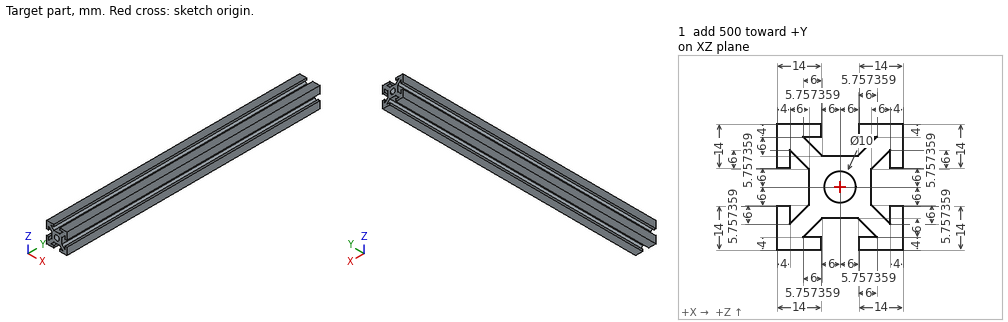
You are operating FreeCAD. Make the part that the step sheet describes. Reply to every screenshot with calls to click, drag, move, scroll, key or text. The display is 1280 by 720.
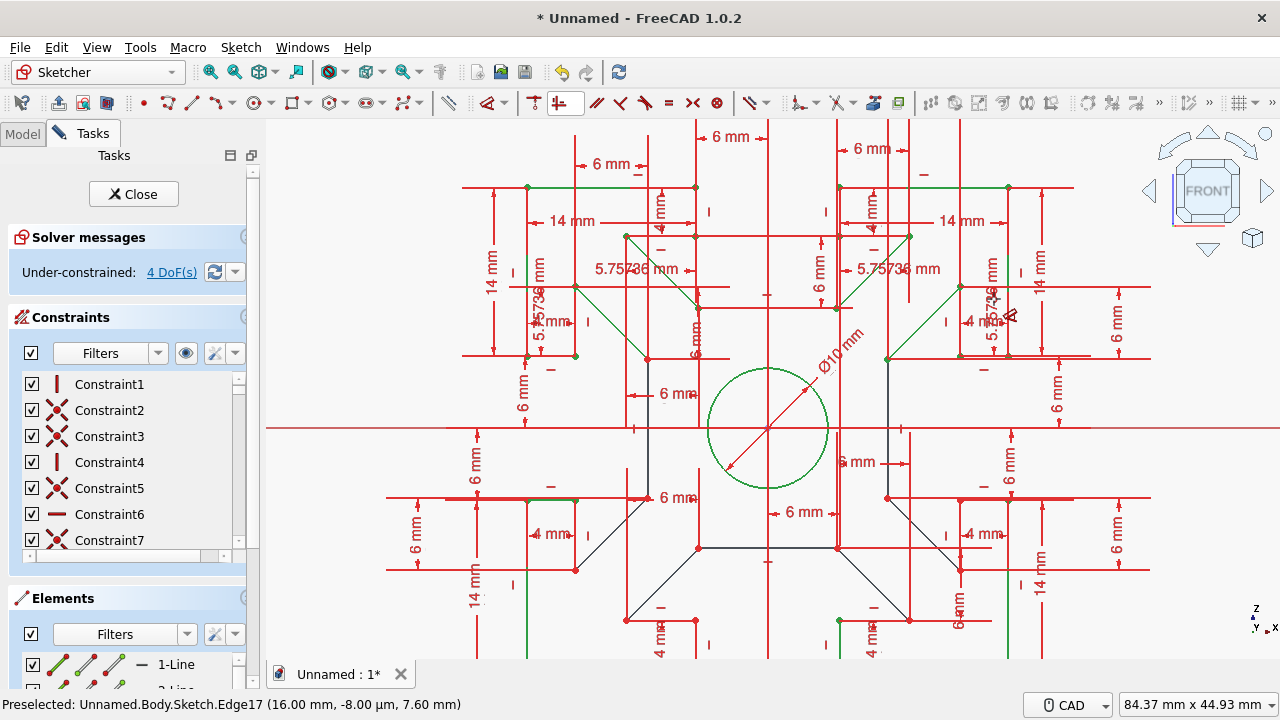
click(960, 549)
click(926, 511)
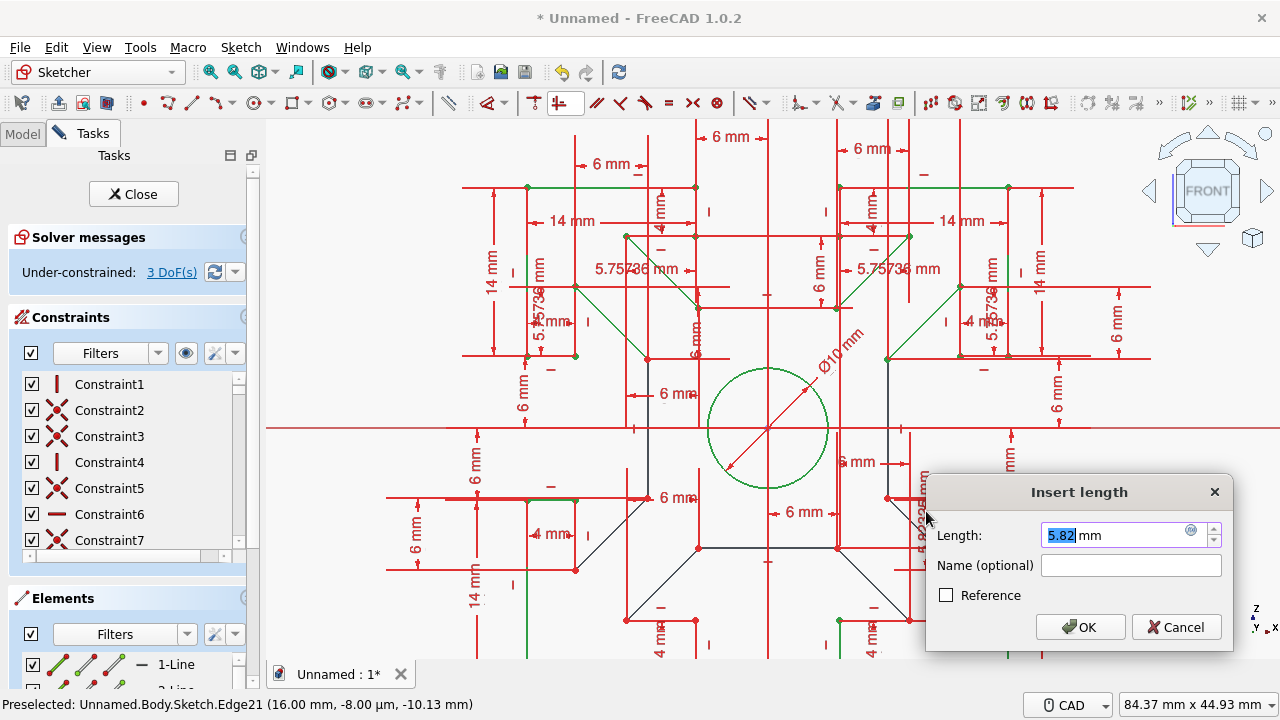
text(5.757359)
key(Return)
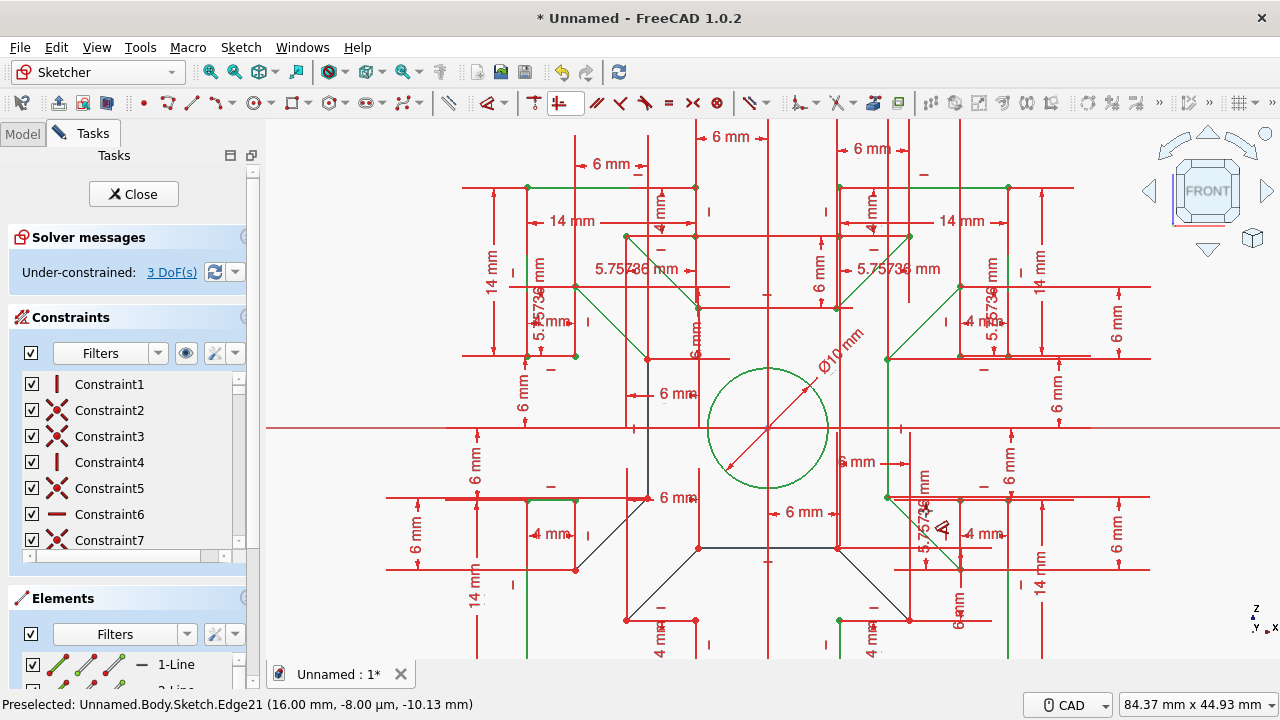
click(861, 621)
click(850, 587)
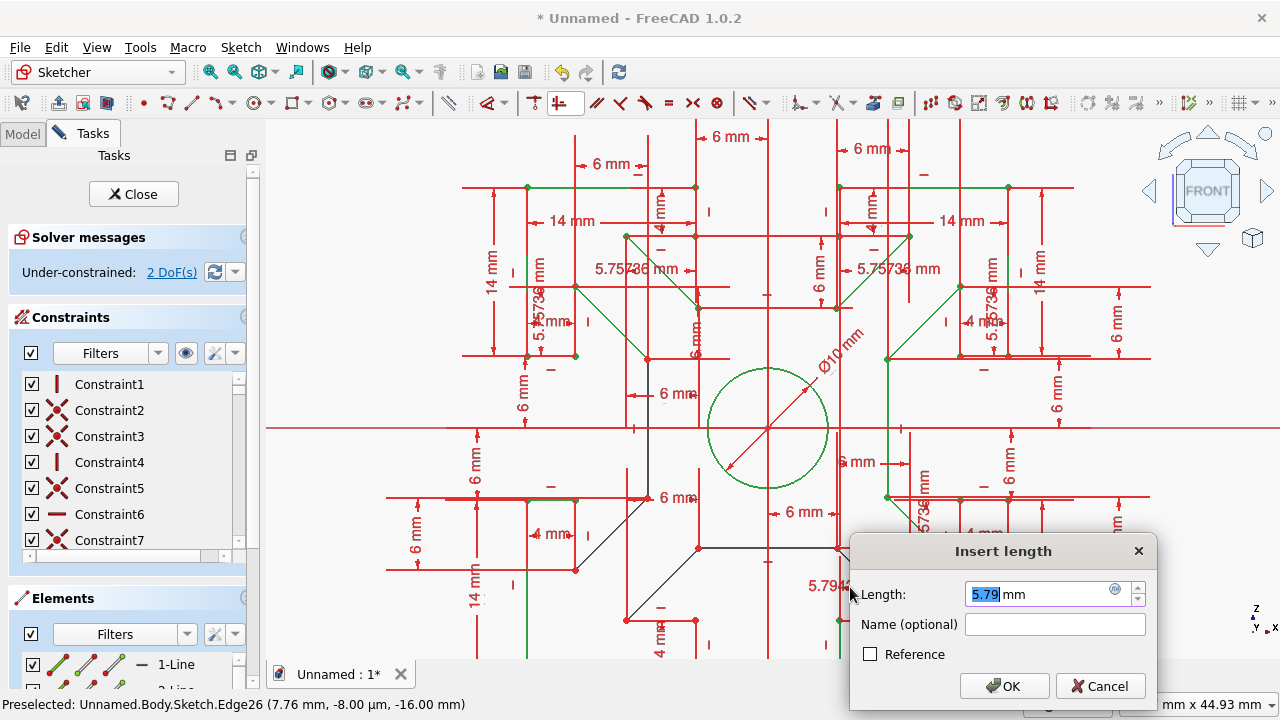
text(5.757359)
key(Return)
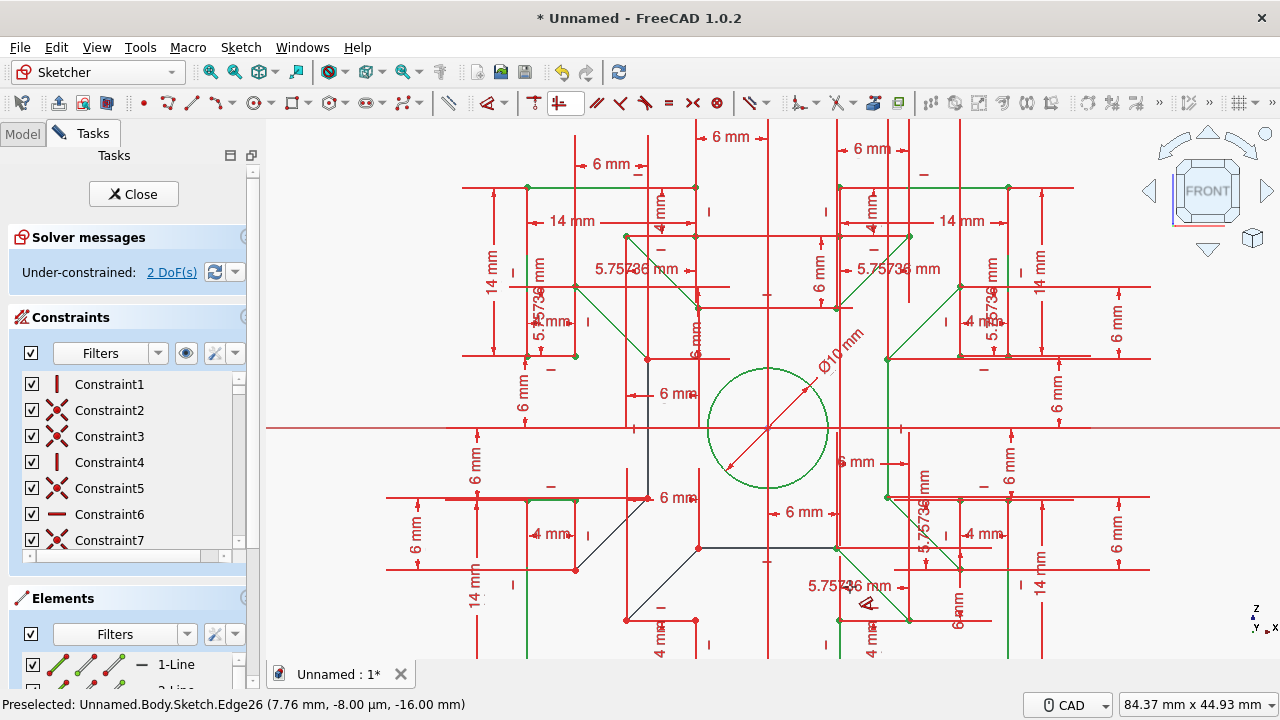
click(647, 621)
click(637, 587)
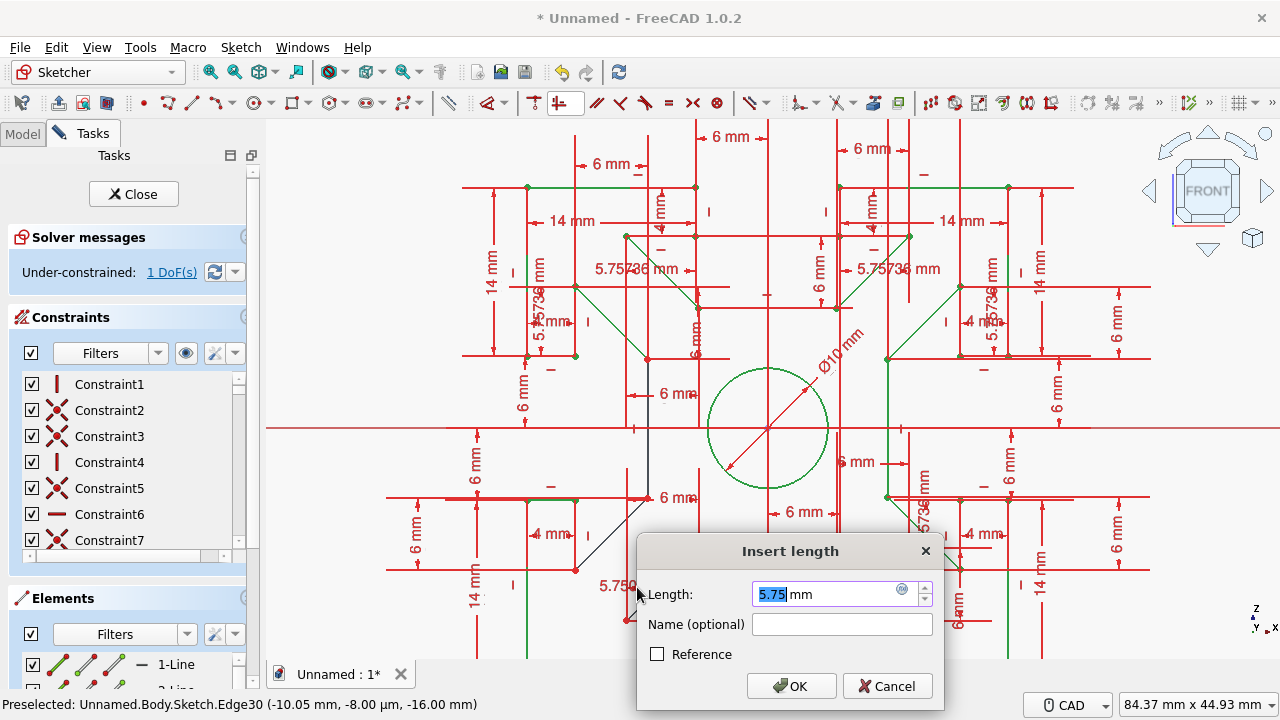
text(5.757359)
key(Return)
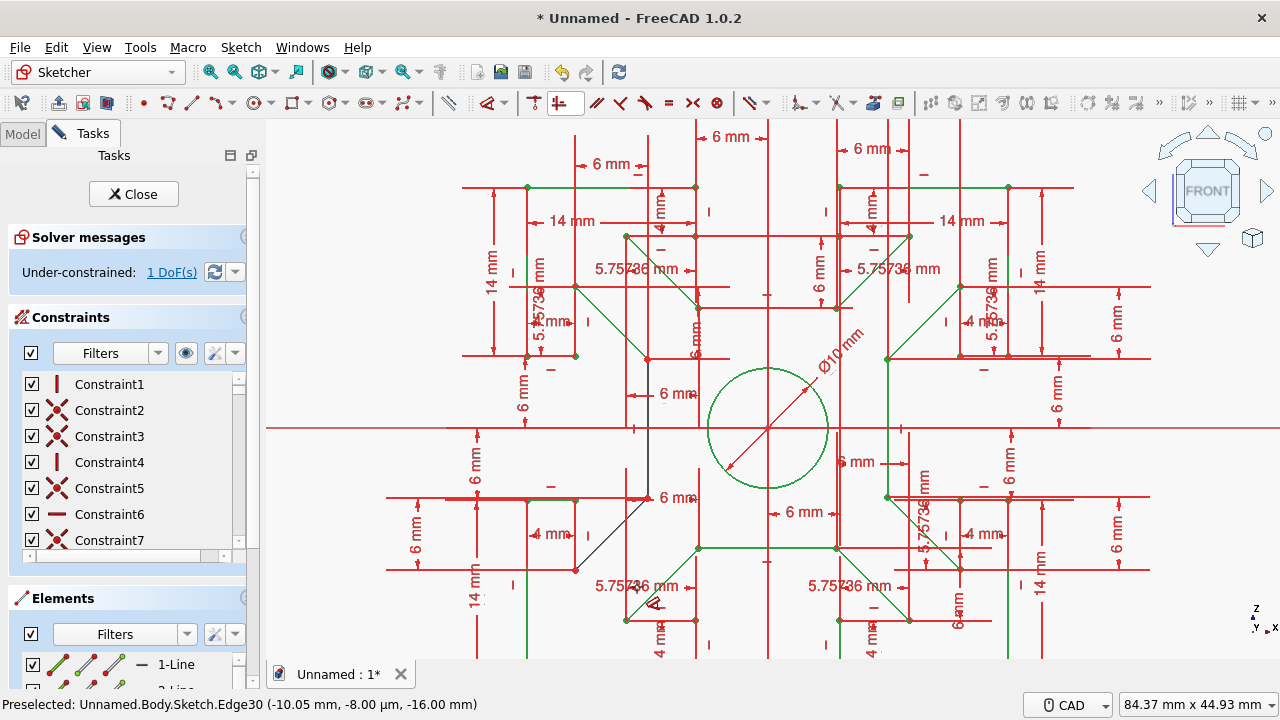
click(575, 521)
click(541, 560)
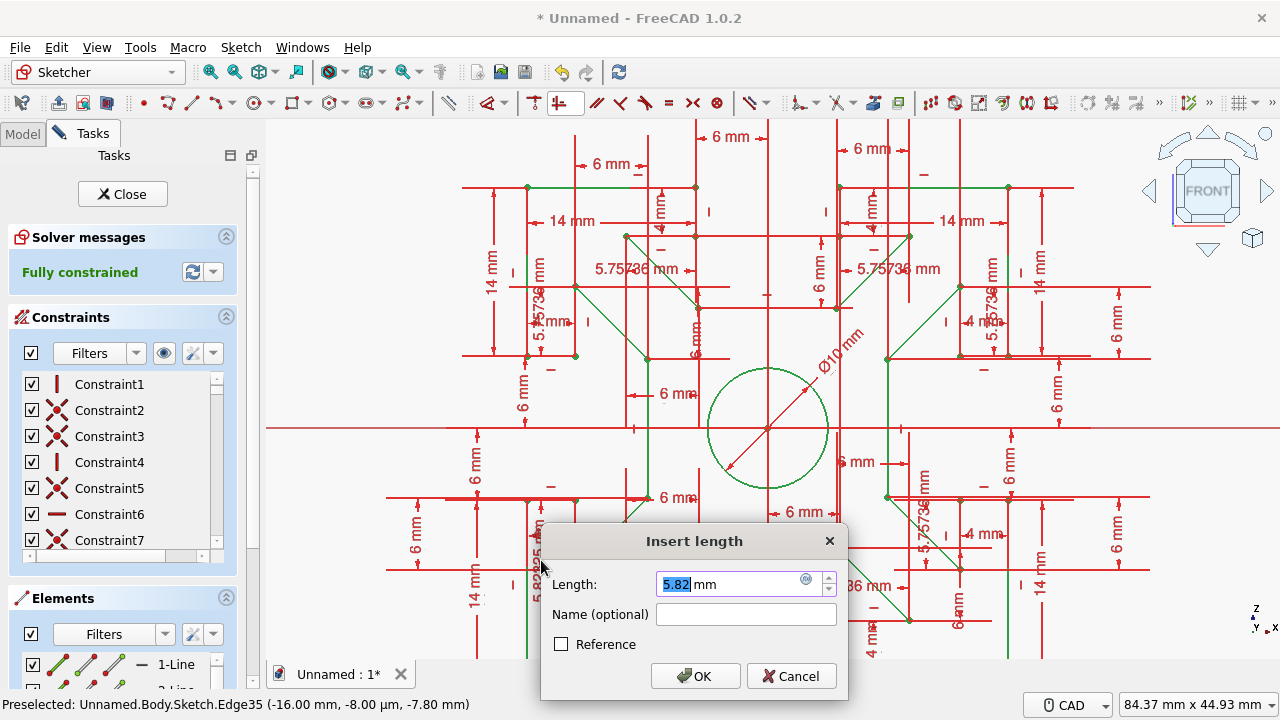
text(5.757359)
key(Return)
key(Escape)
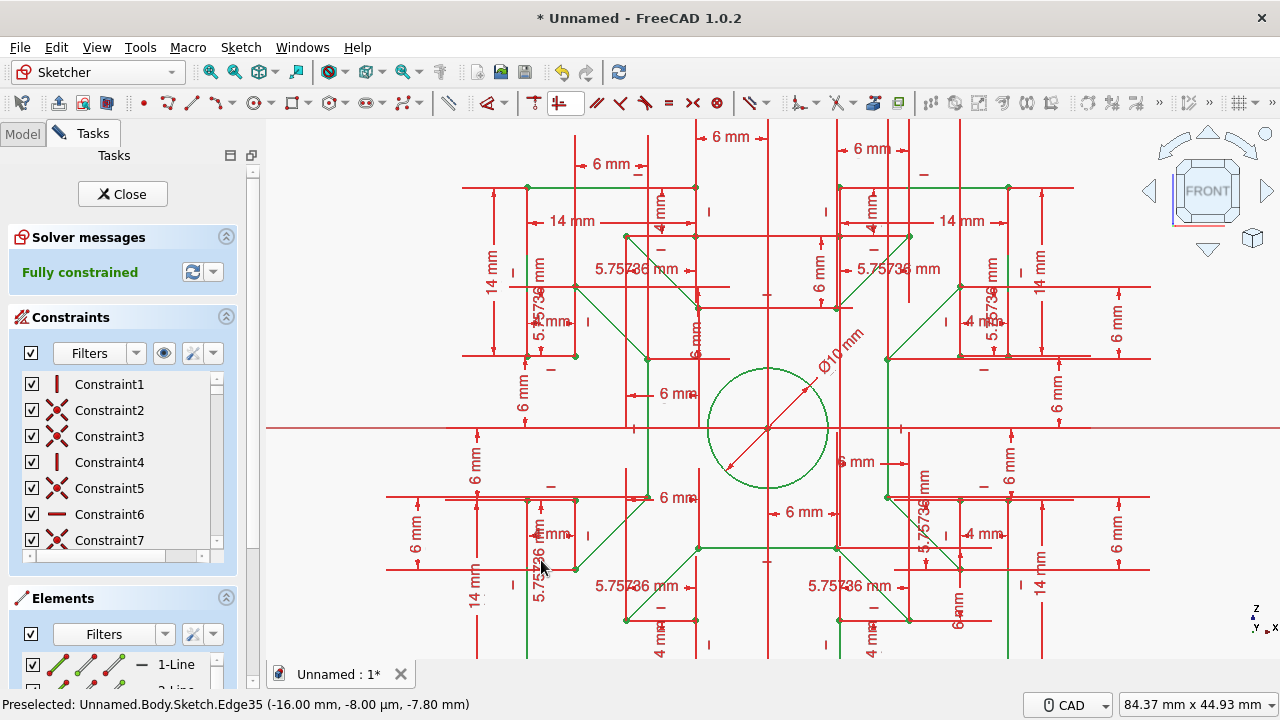
click(123, 194)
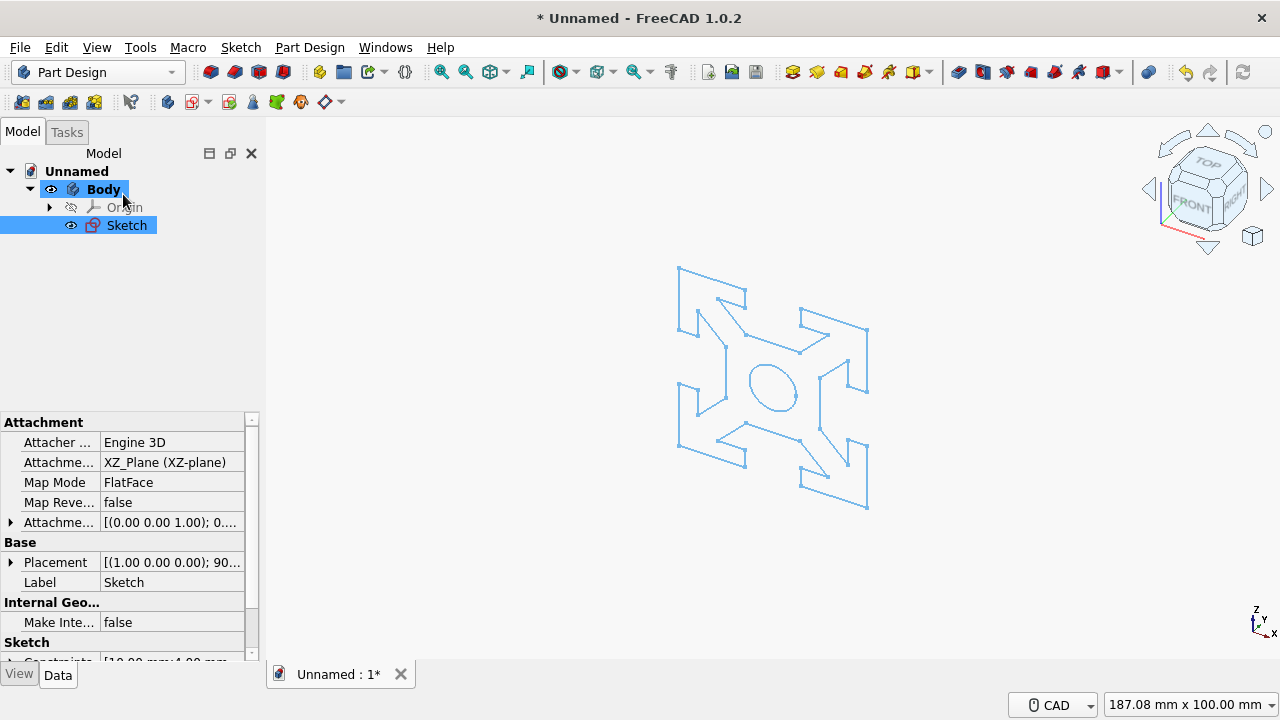
click(794, 72)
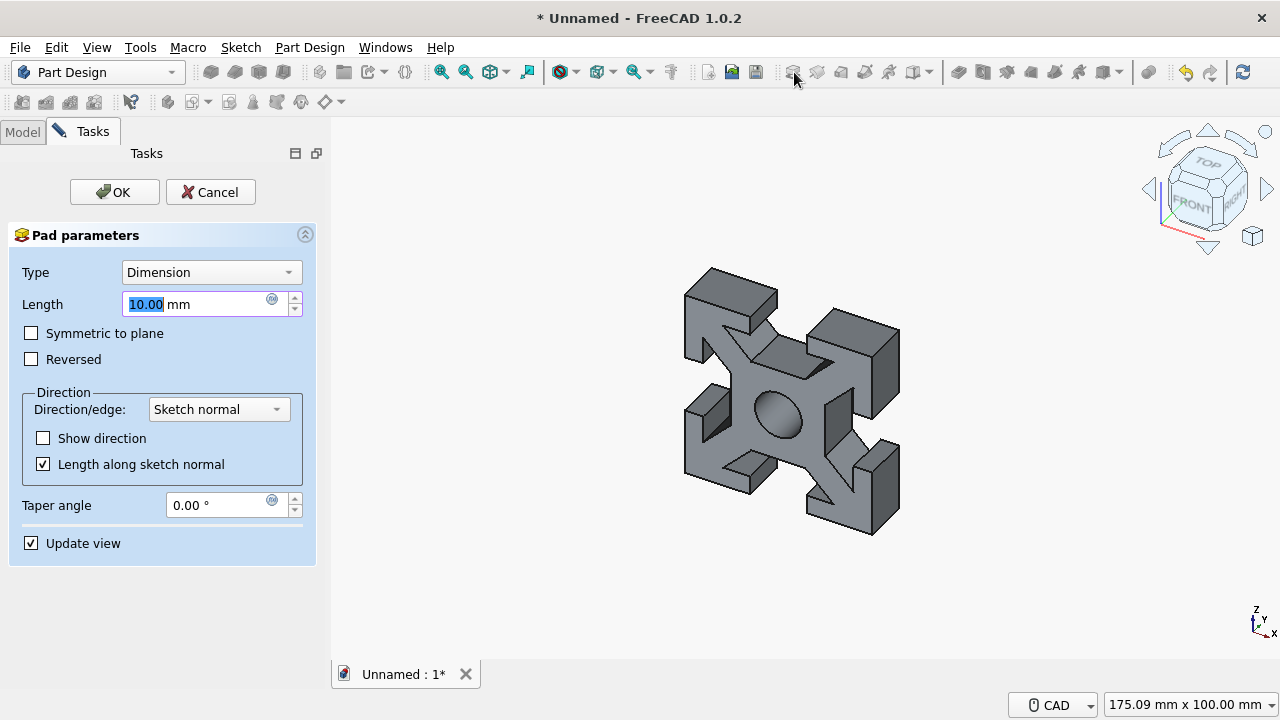
text(500)
key(Tab)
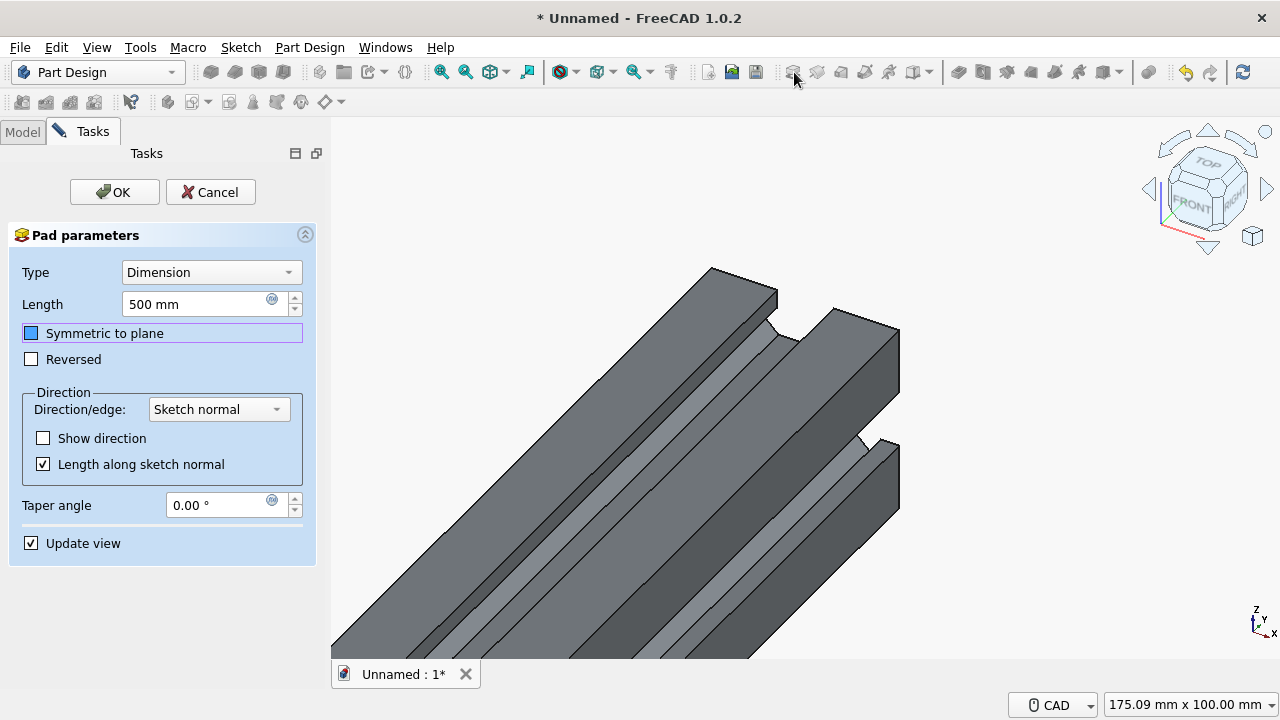
click(30, 359)